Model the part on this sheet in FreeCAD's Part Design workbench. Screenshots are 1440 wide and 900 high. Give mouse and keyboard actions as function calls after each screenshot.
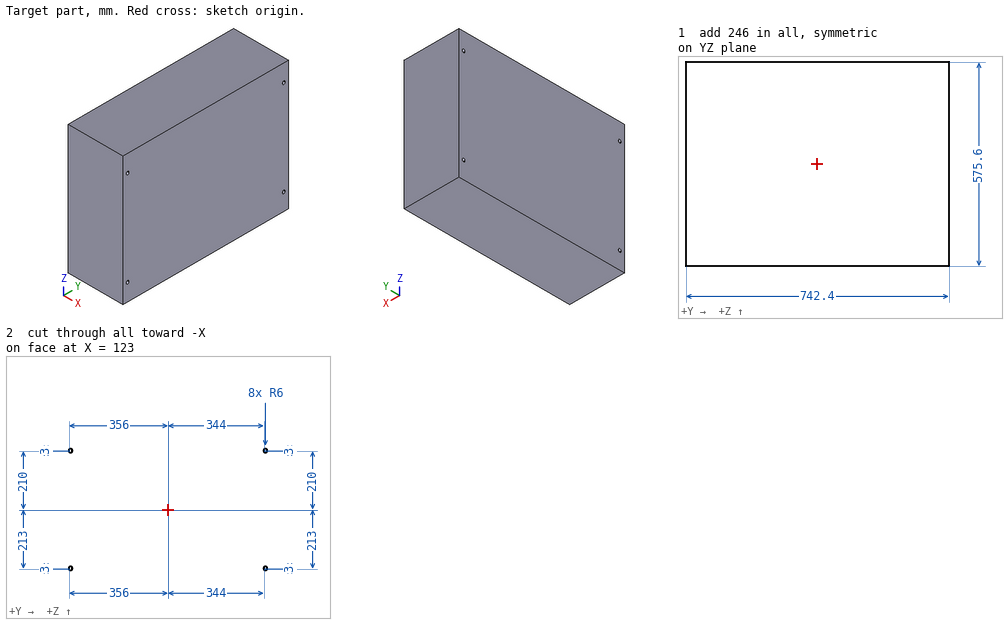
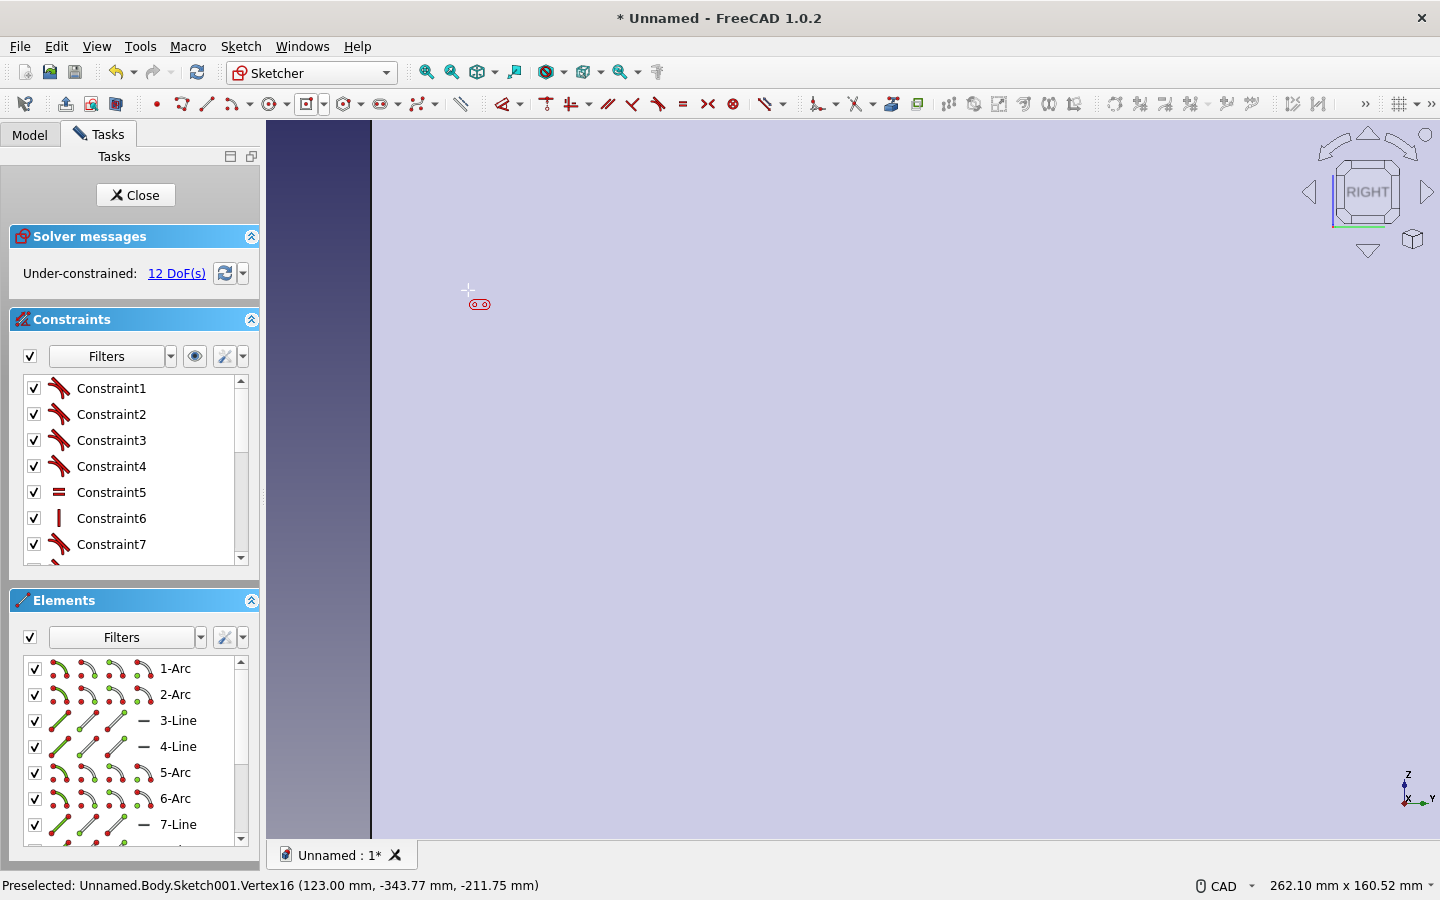
scroll(468, 289, down, 8)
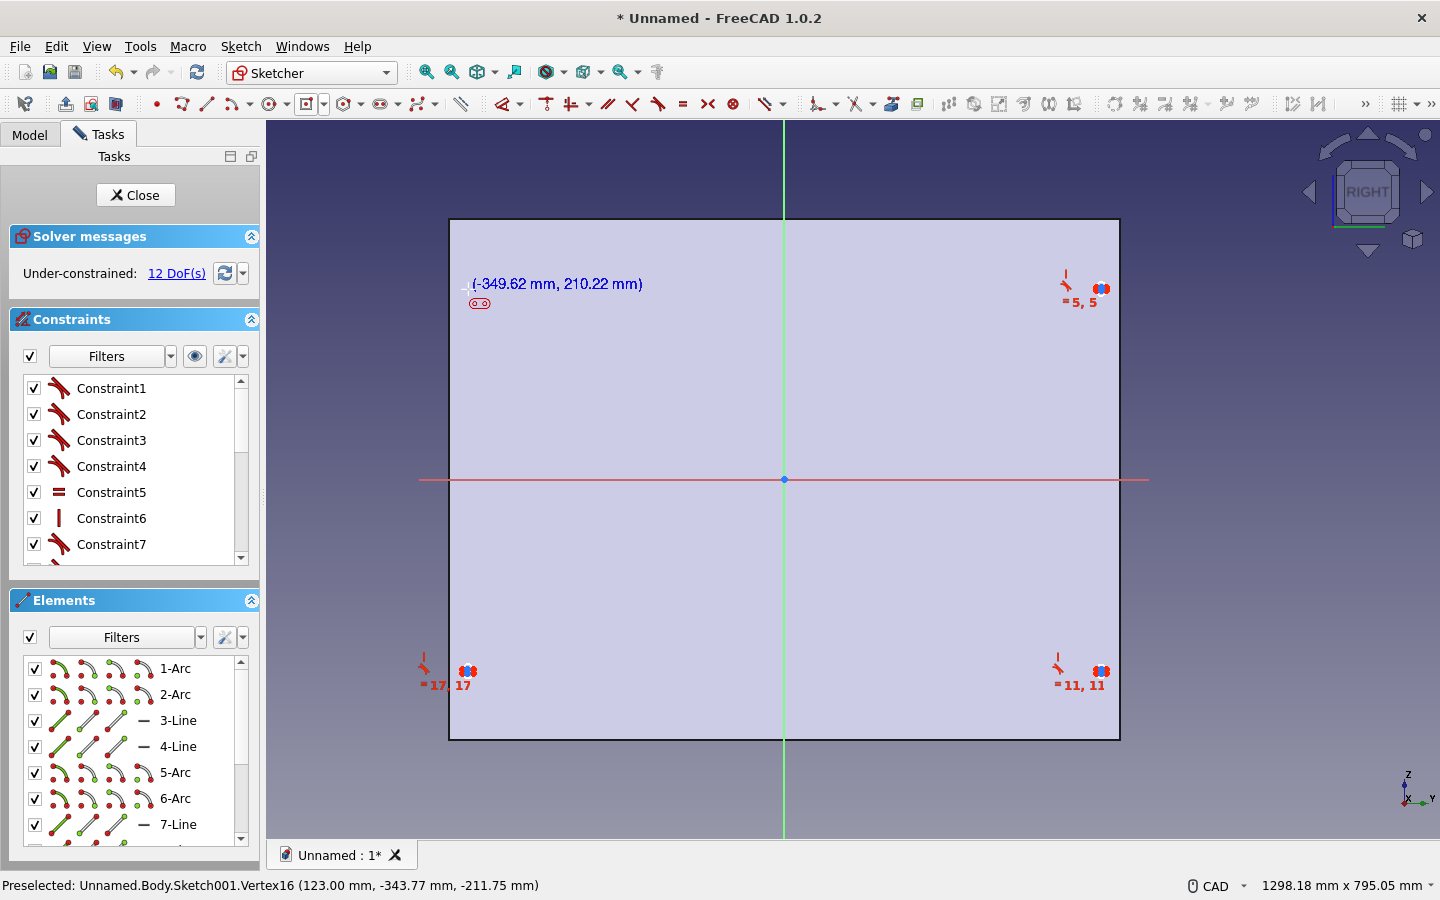
click(468, 290)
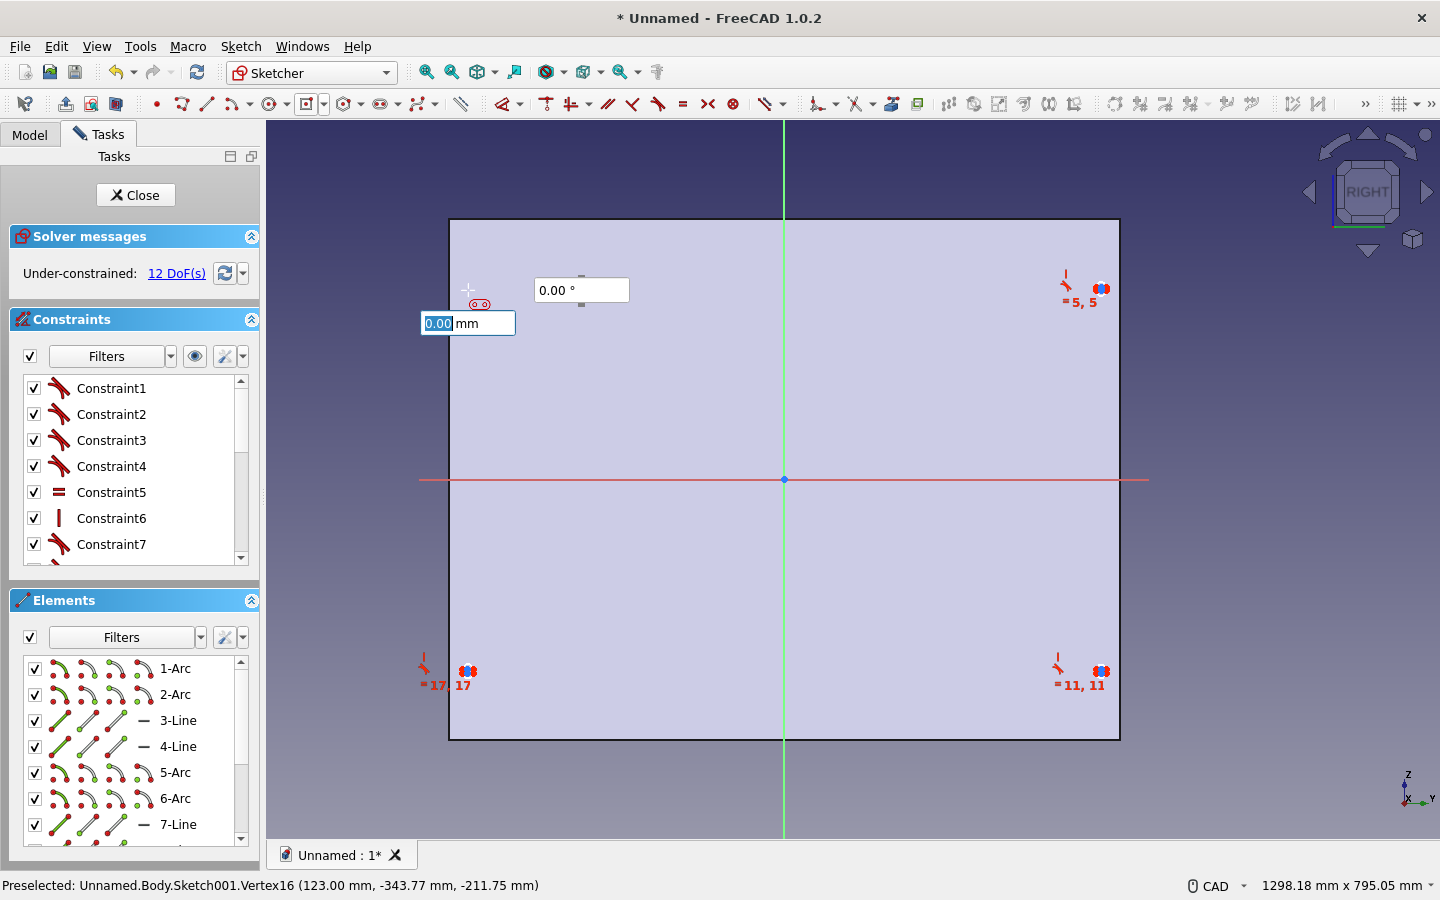
scroll(468, 287, up, 9)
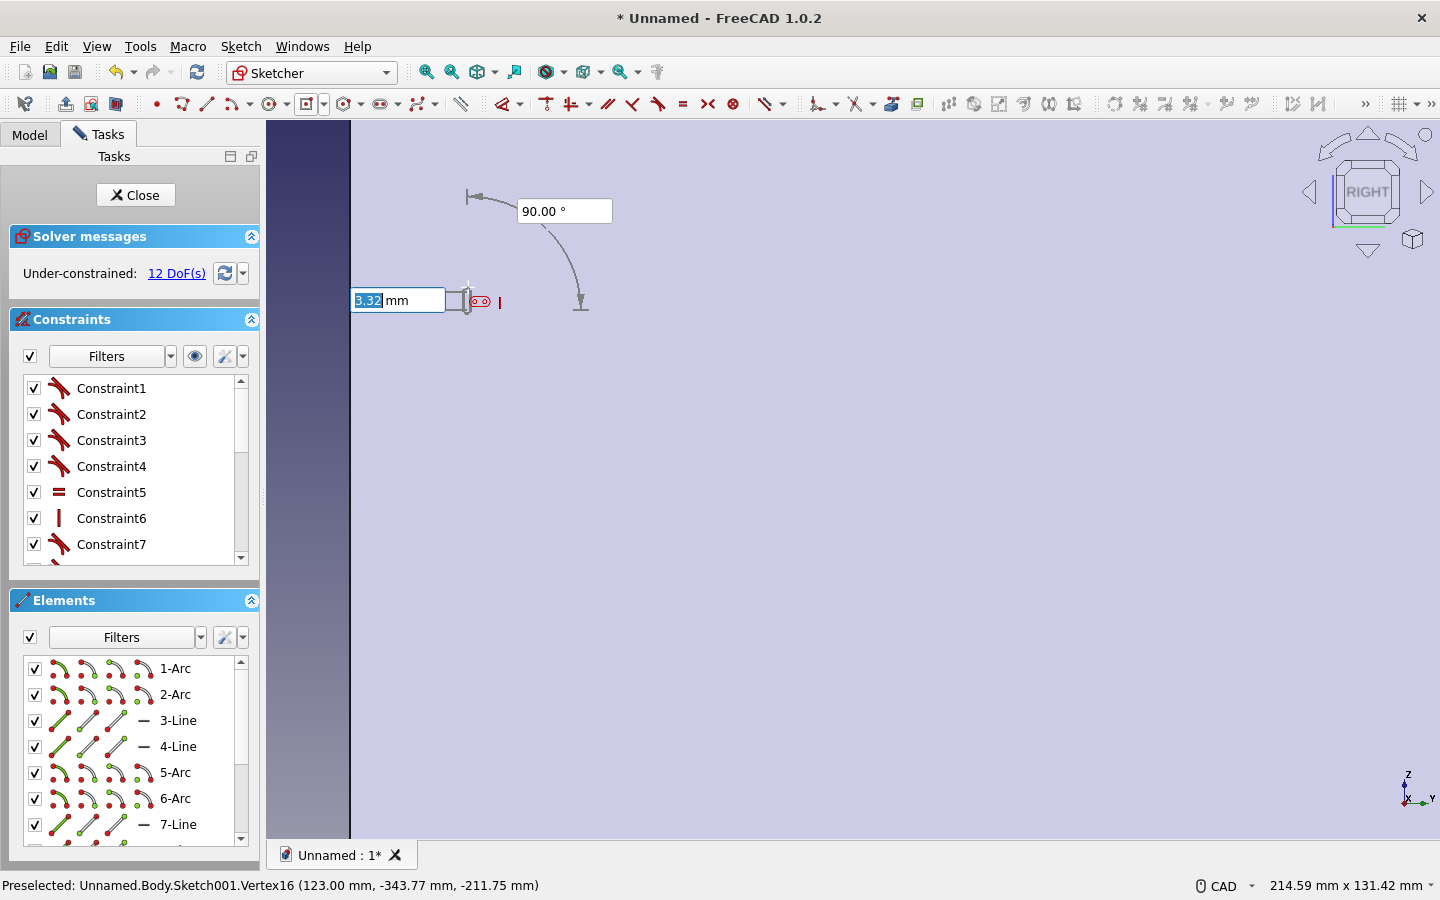
click(467, 285)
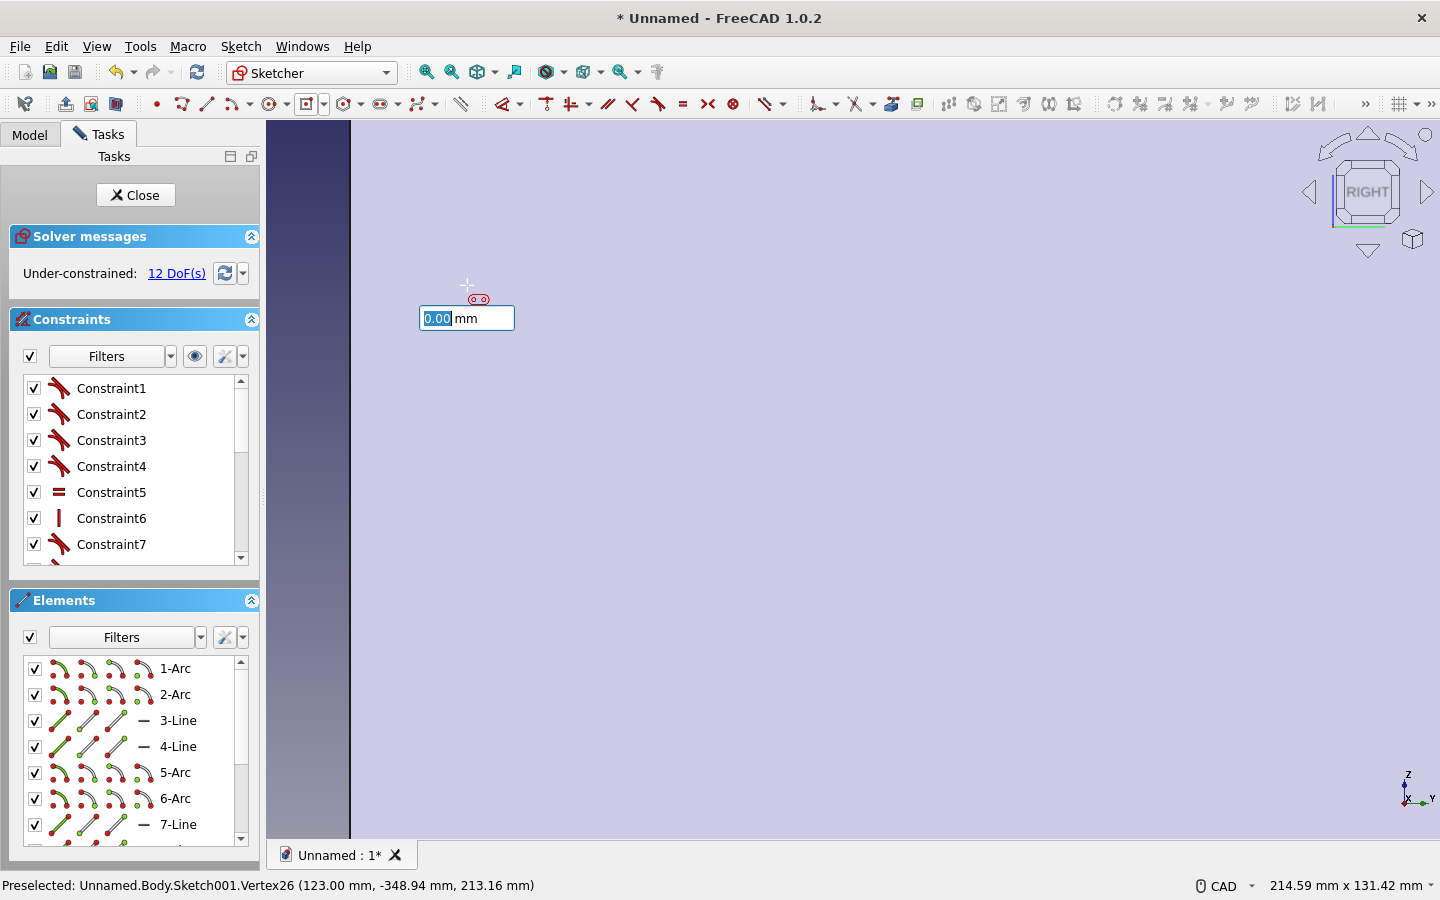
click(499, 293)
key(Escape)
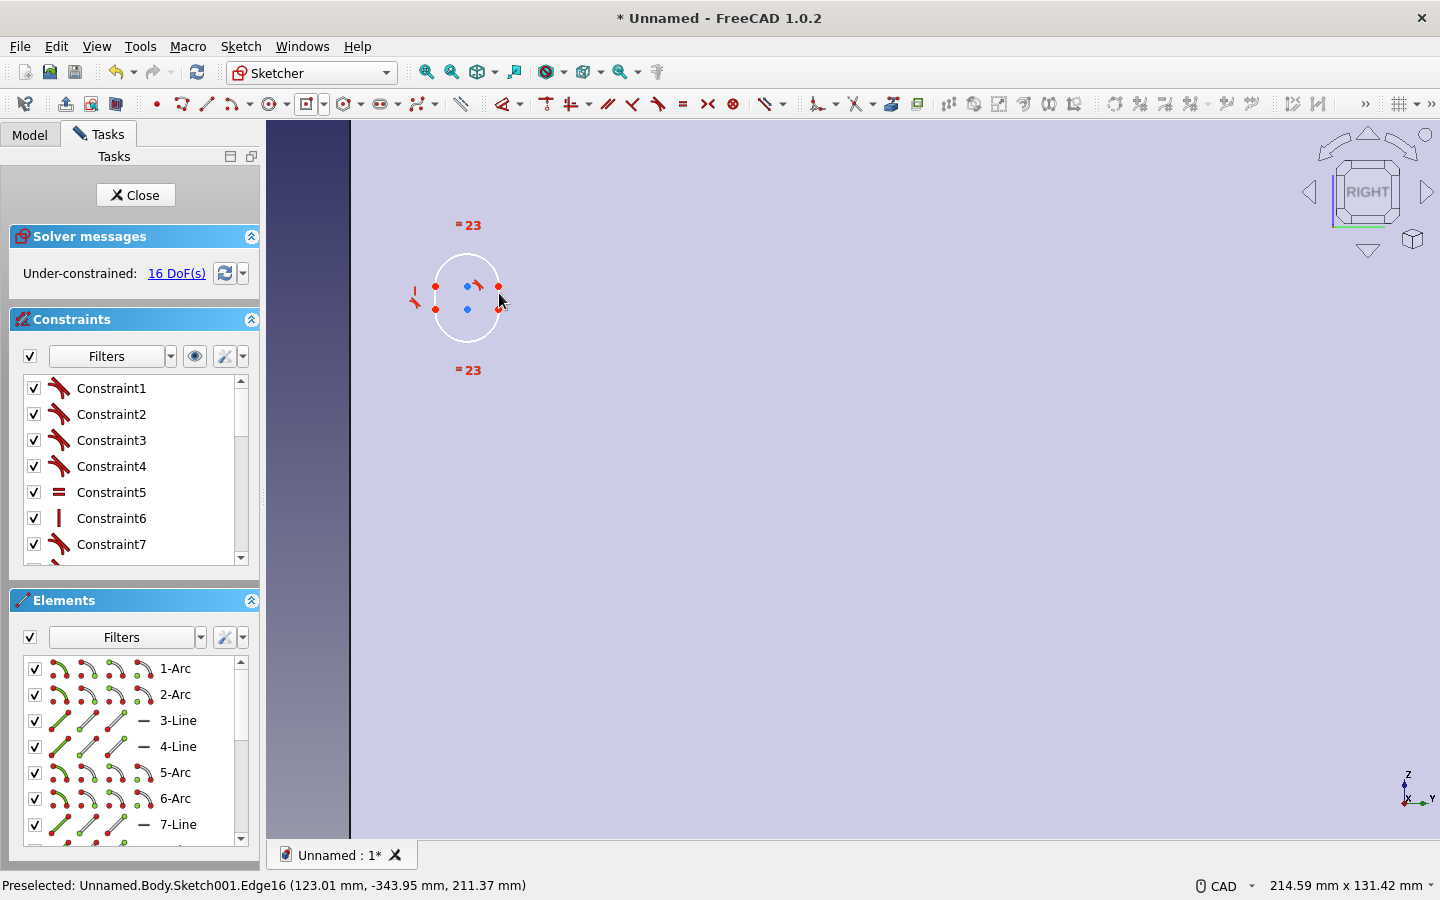
scroll(468, 287, down, 9)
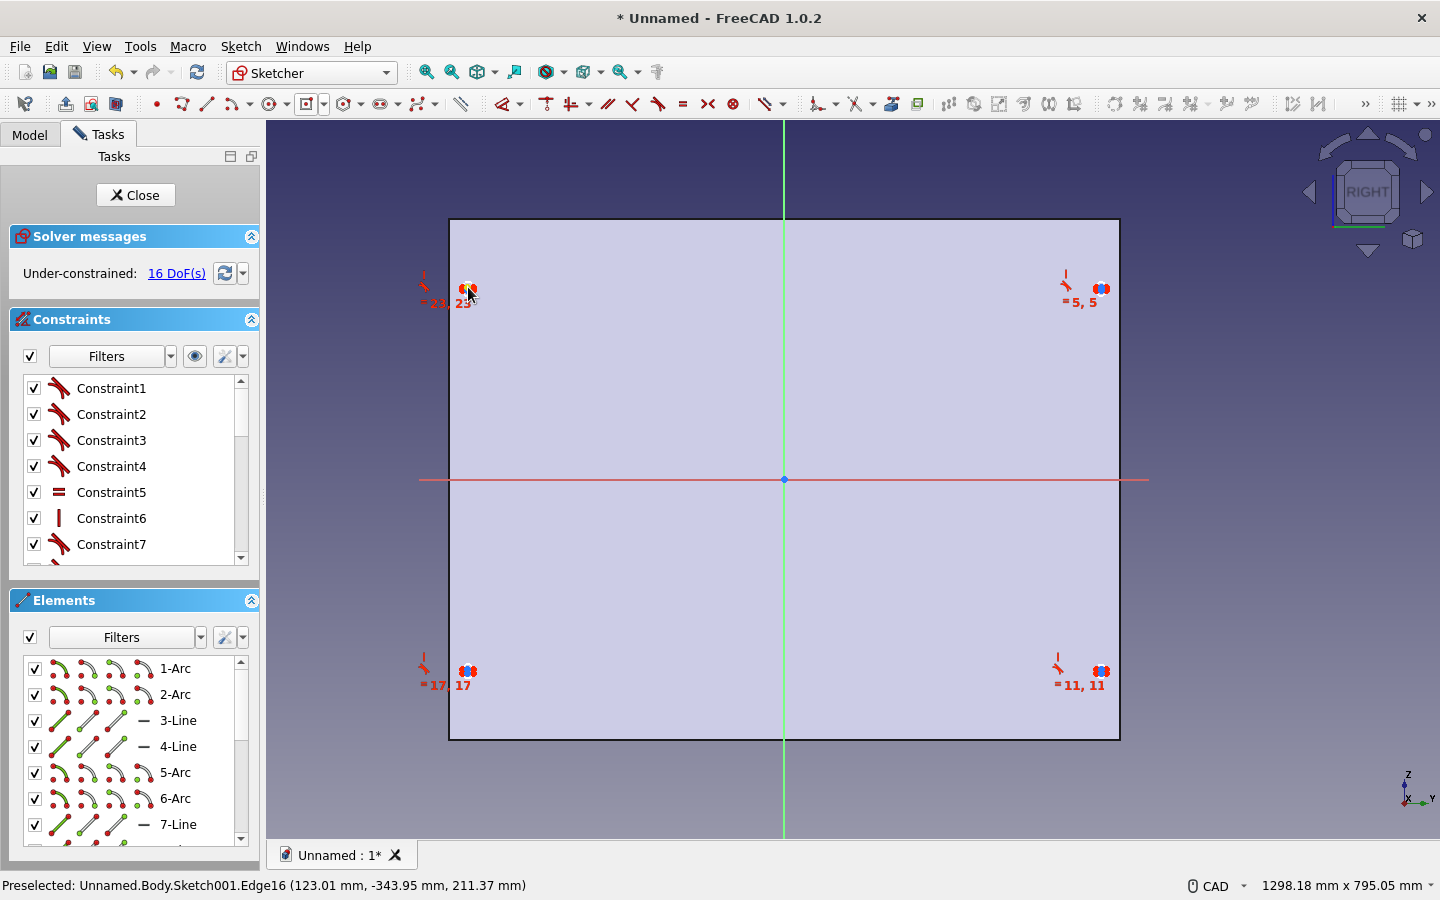
scroll(1098, 295, up, 6)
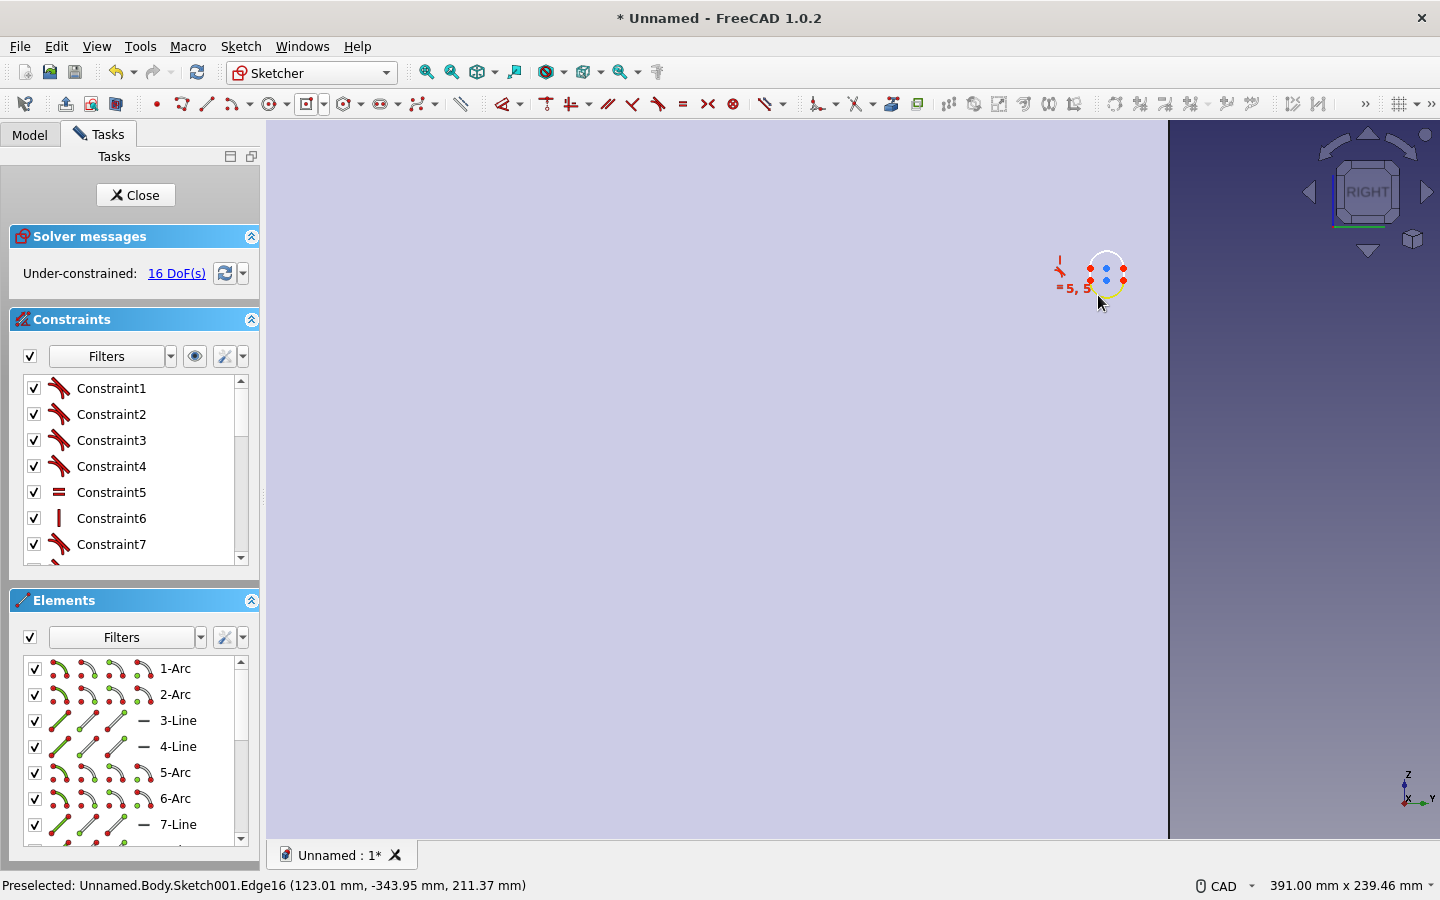
click(1097, 295)